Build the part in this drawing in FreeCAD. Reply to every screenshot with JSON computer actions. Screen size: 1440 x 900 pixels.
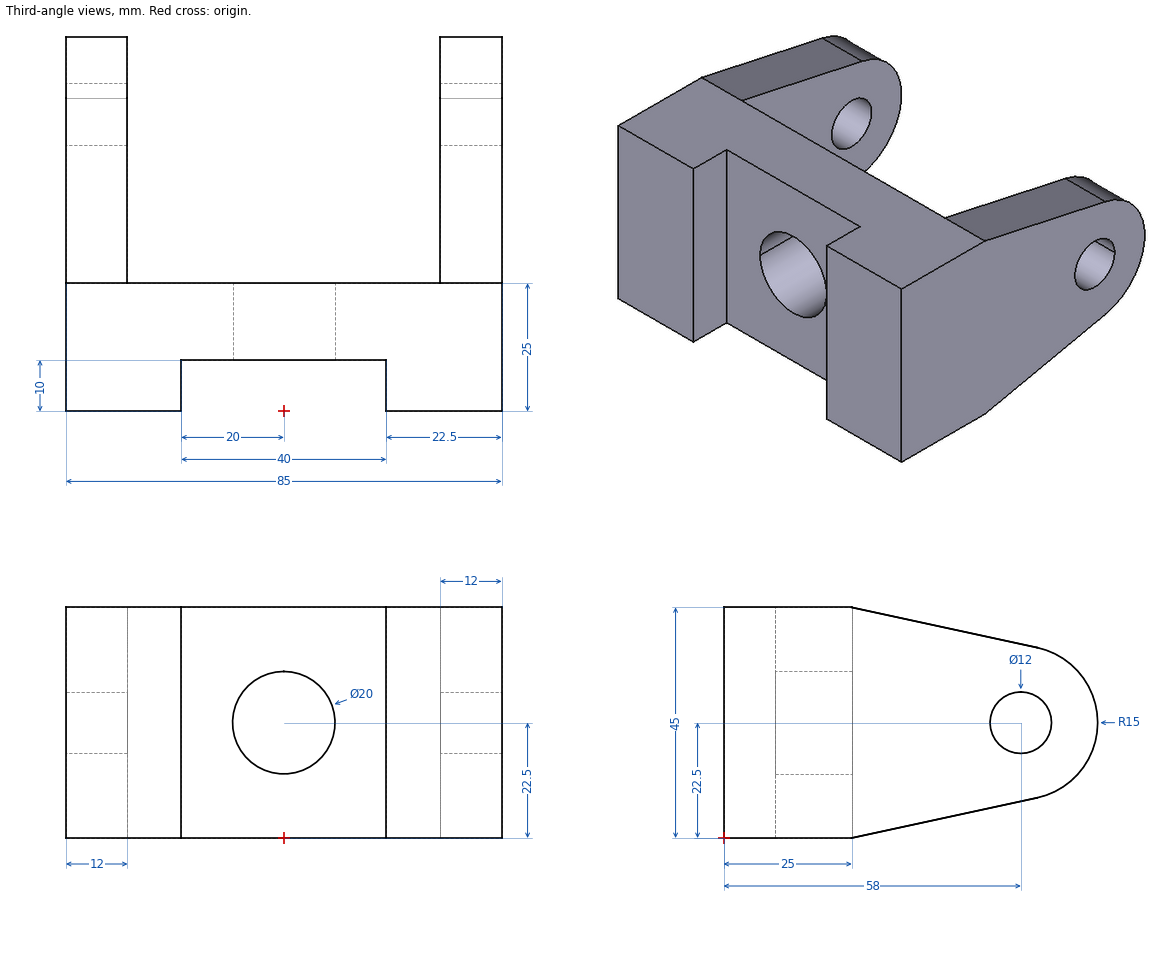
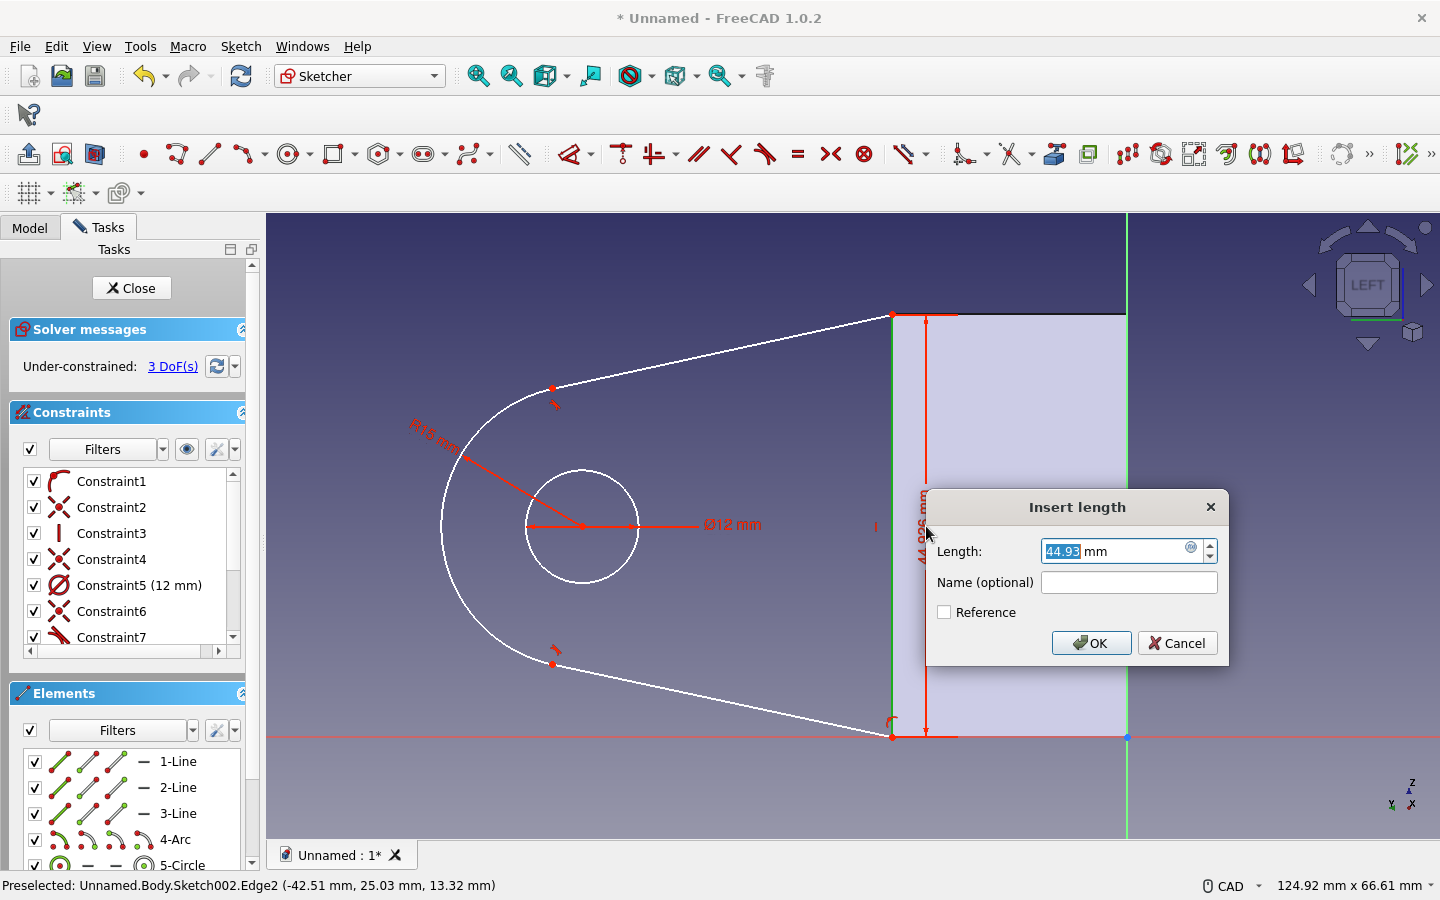
{"action": "type", "text": "45"}
{"action": "key", "text": "Return"}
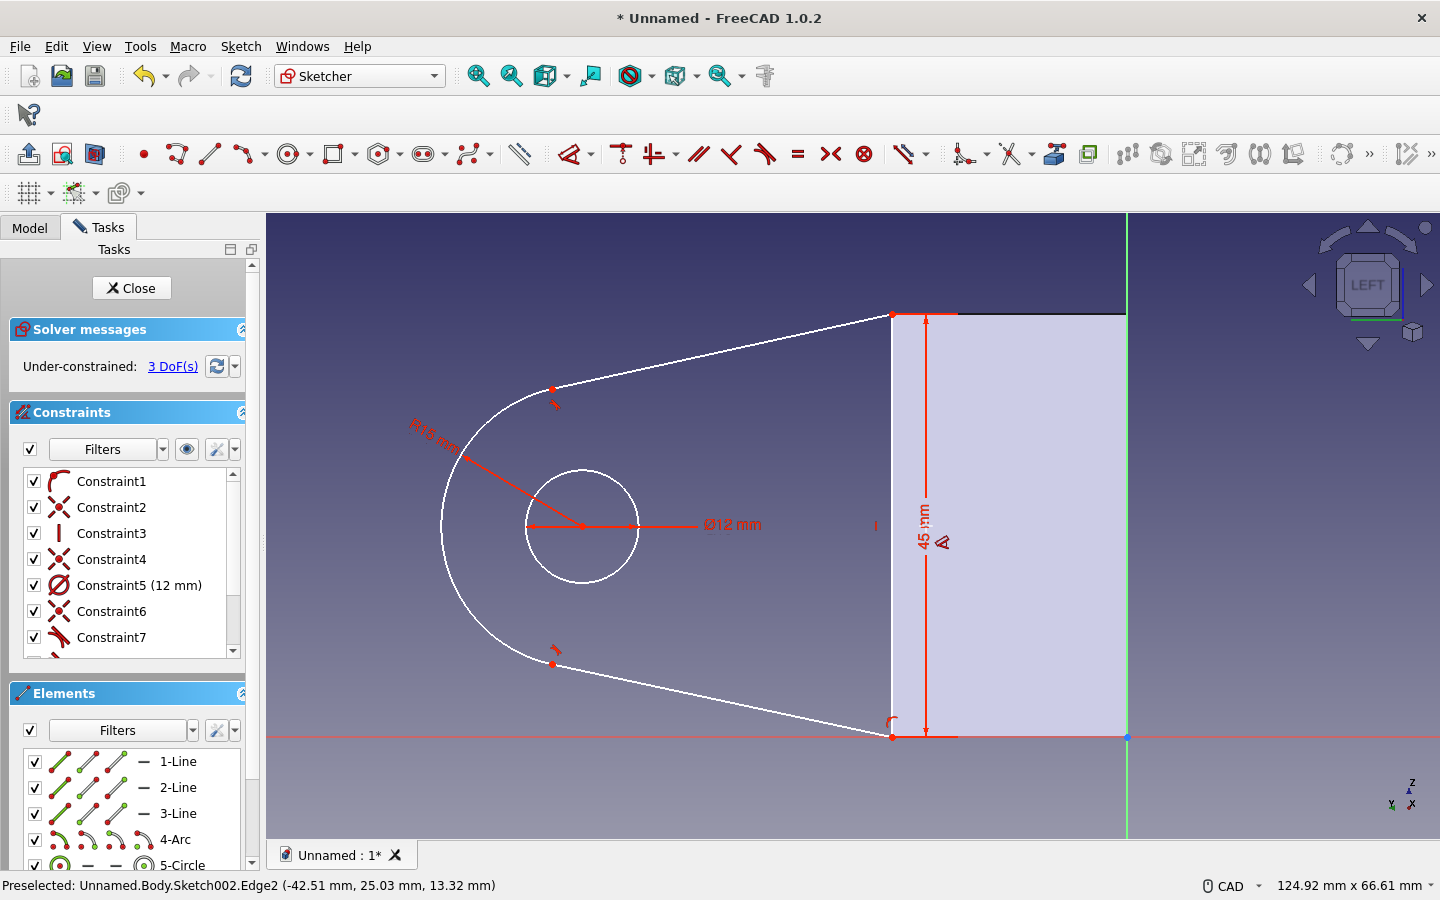
{"action": "left_click", "coordinate": [582, 527]}
{"action": "left_click", "coordinate": [855, 771]}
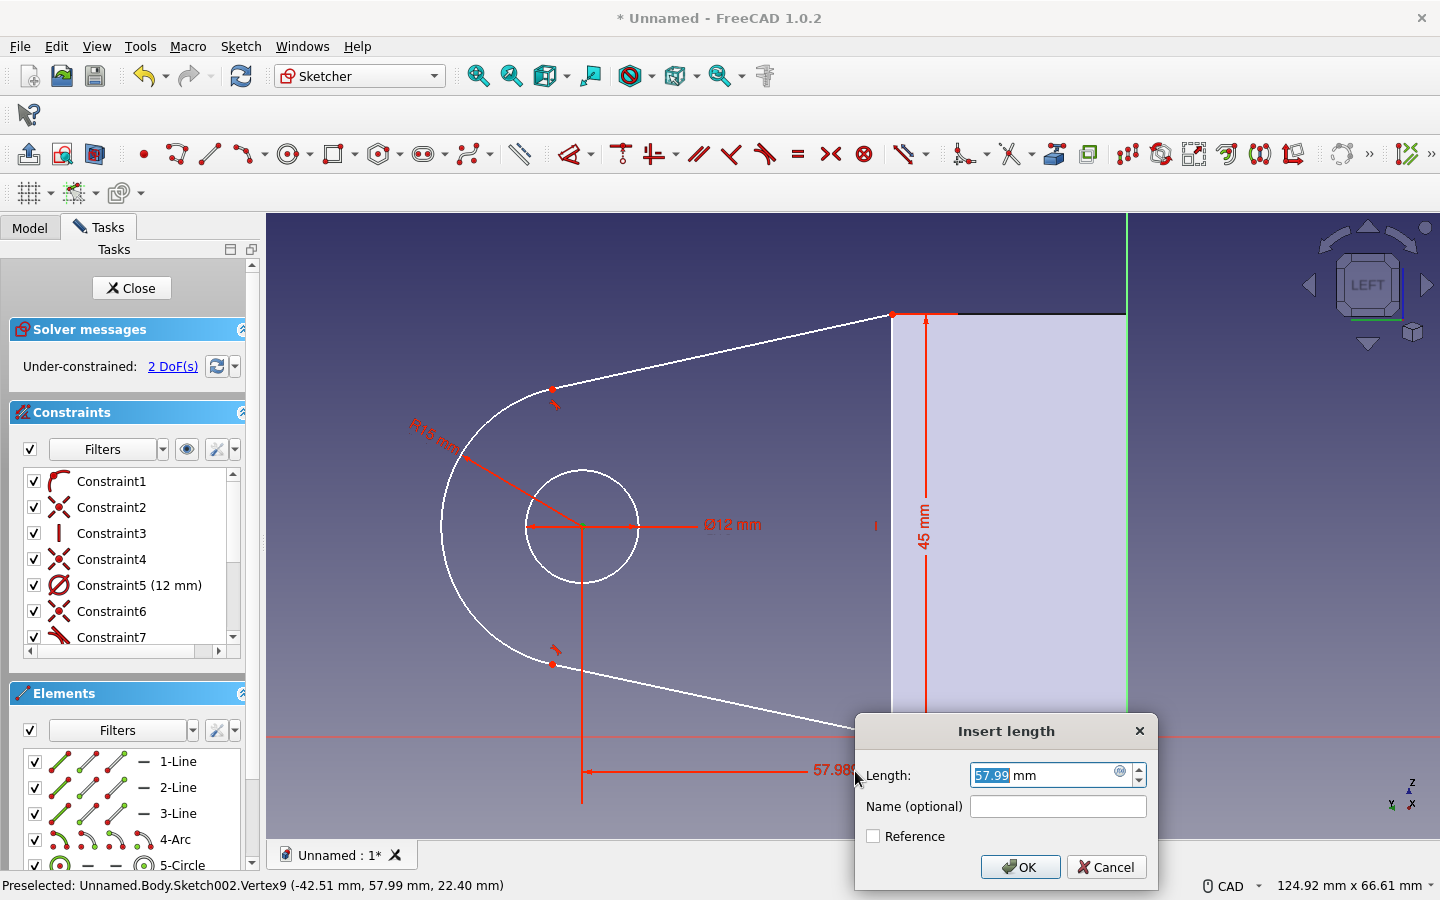
{"action": "type", "text": "58"}
{"action": "key", "text": "Return"}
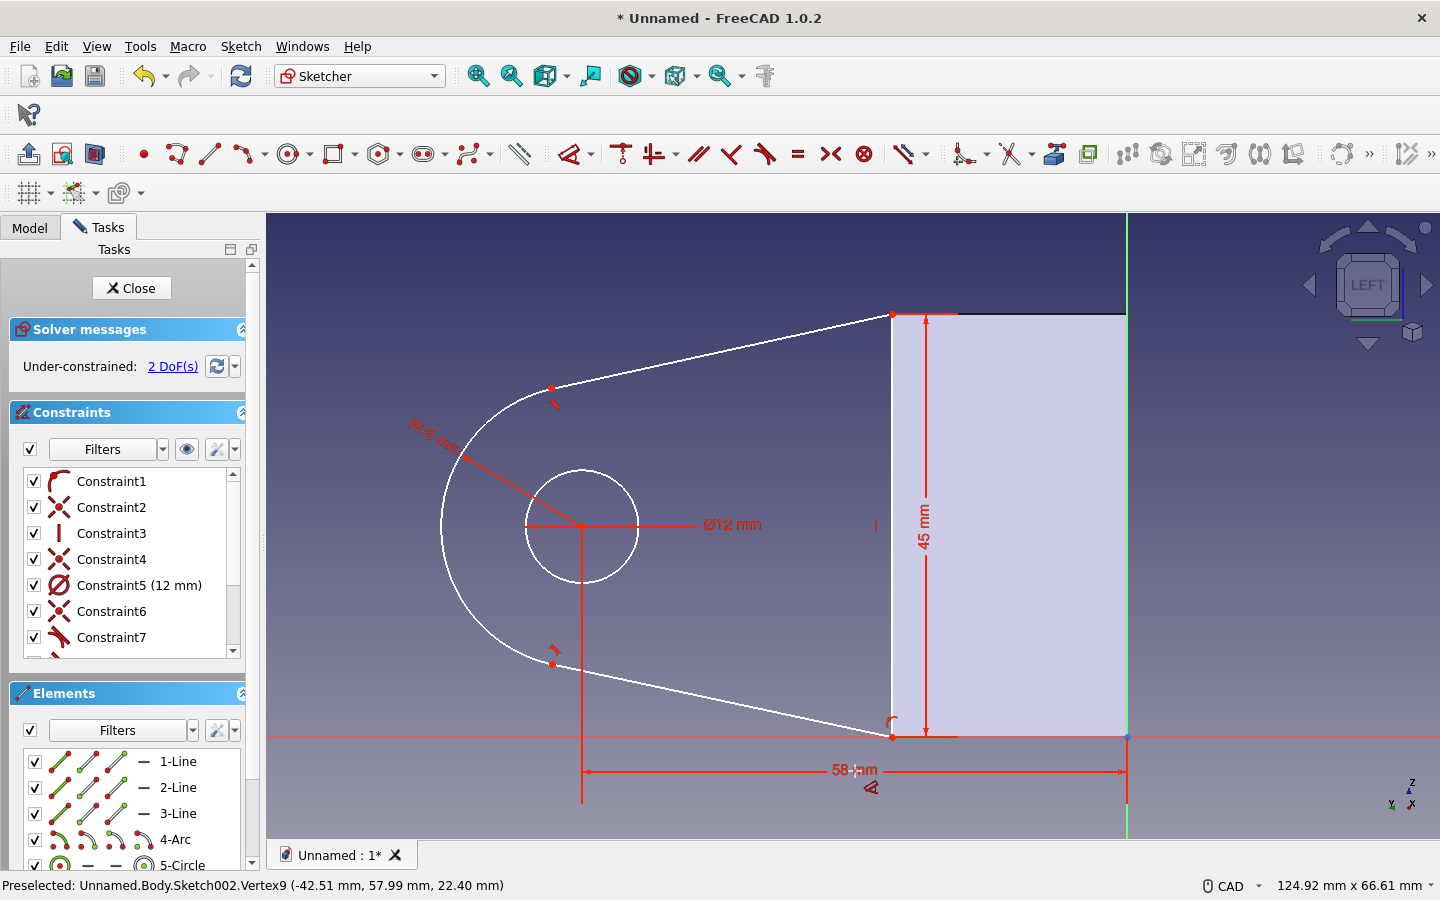
{"action": "left_click", "coordinate": [892, 737]}
{"action": "left_click", "coordinate": [1010, 771]}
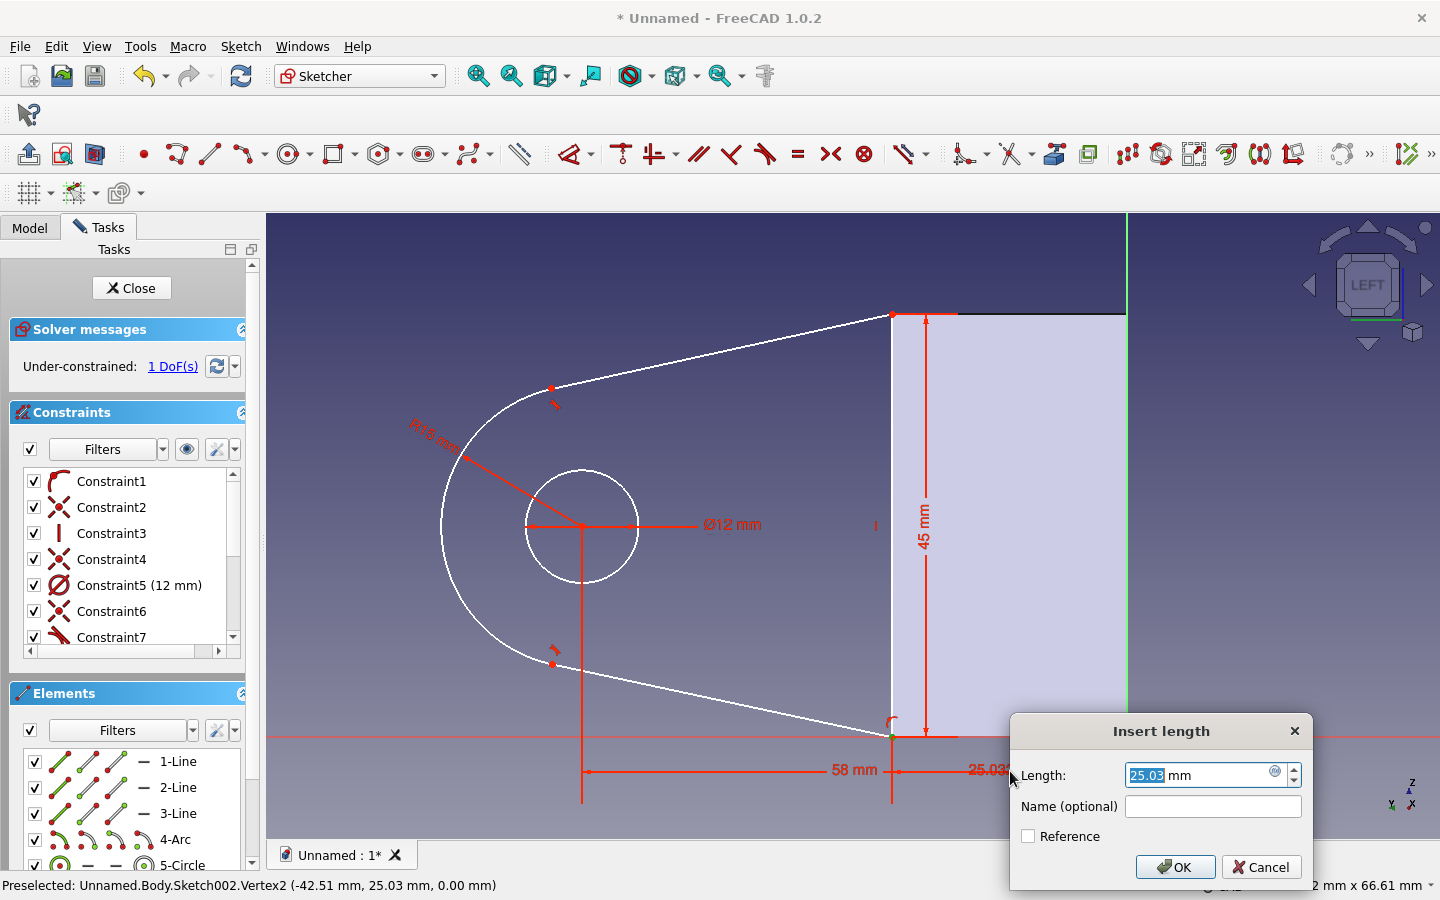
{"action": "type", "text": "25"}
{"action": "key", "text": "Return"}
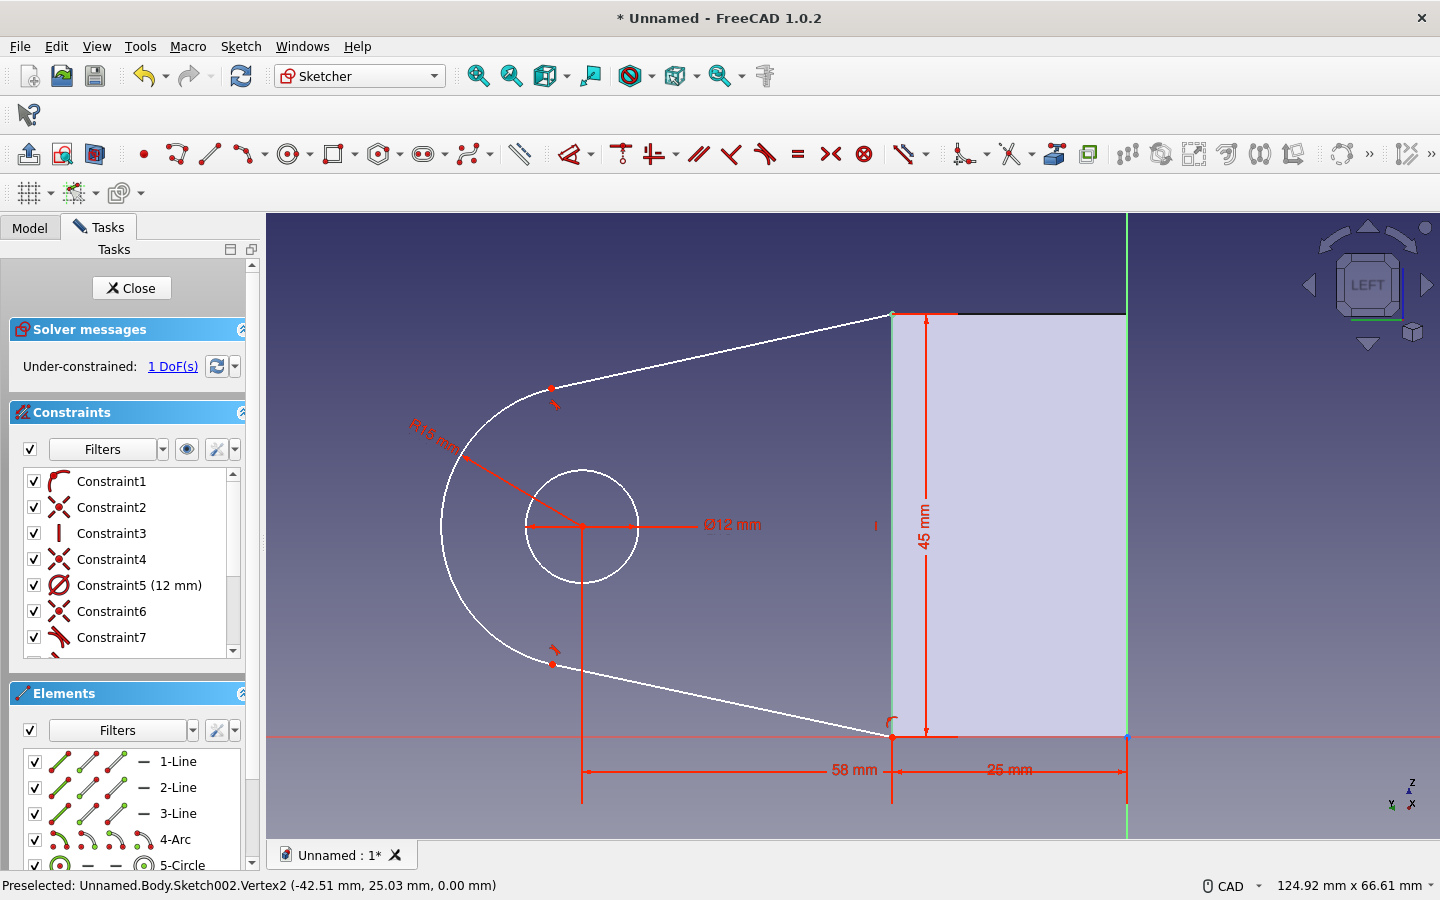
{"action": "left_click", "coordinate": [582, 527]}
{"action": "left_click", "coordinate": [1161, 632]}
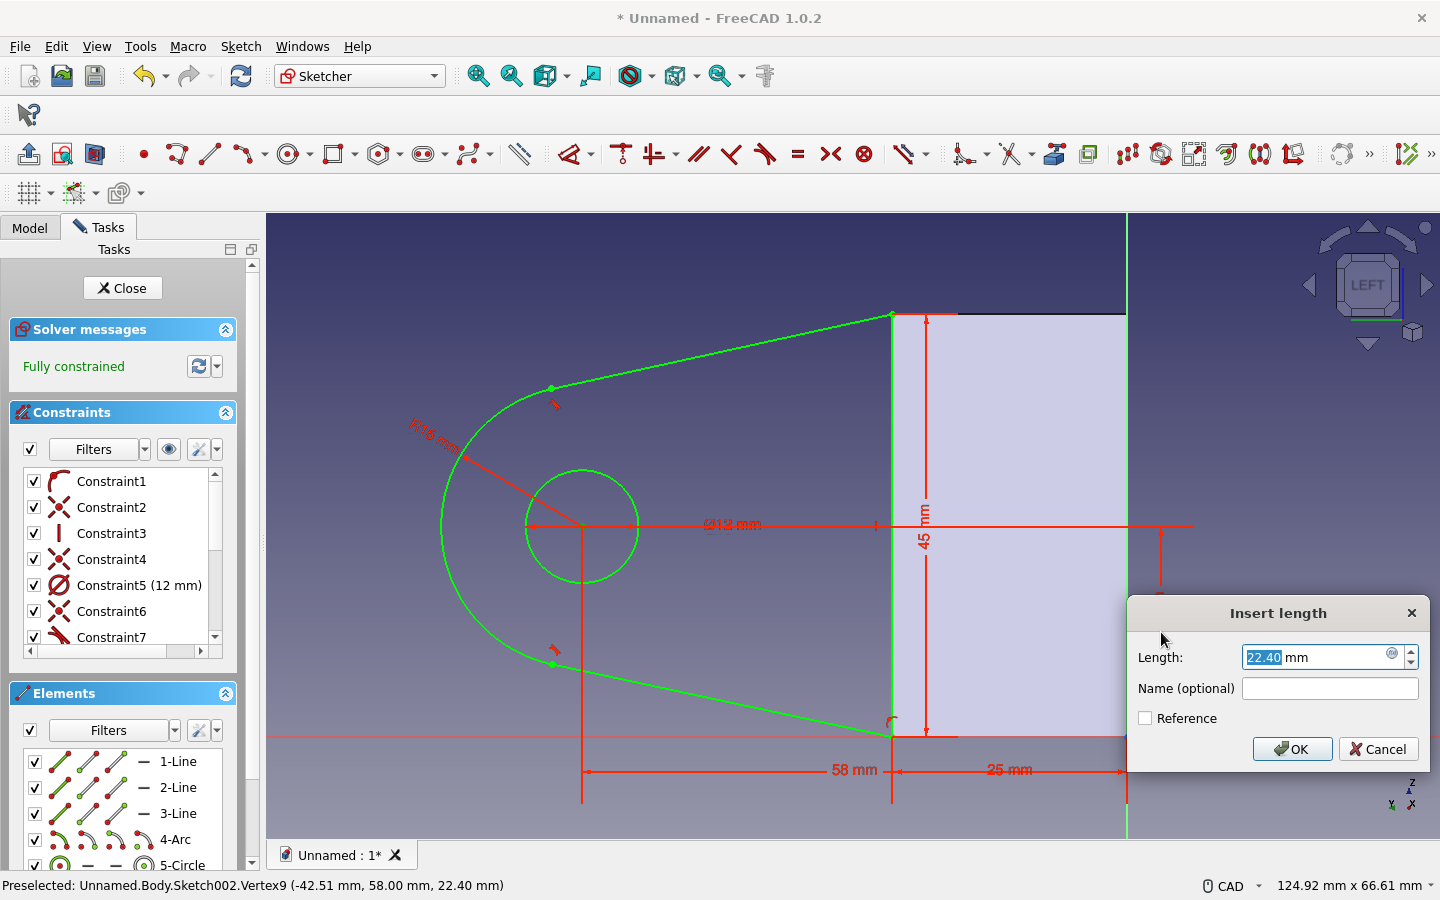
{"action": "type", "text": "22.5"}
{"action": "key", "text": "Return"}
{"action": "key", "text": "Escape"}